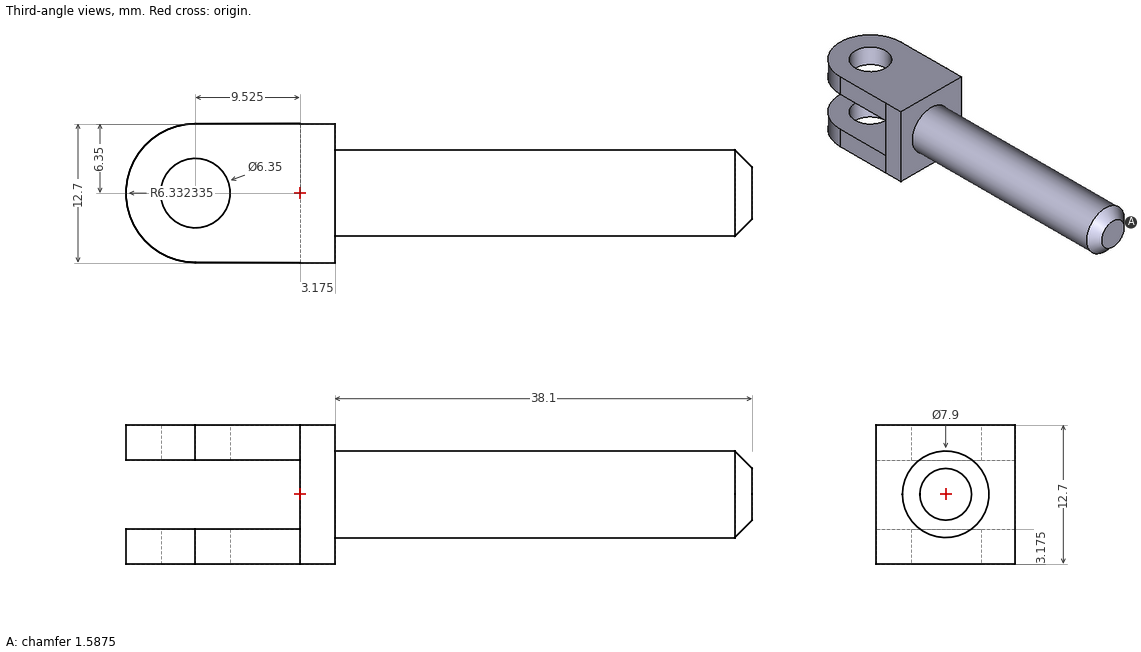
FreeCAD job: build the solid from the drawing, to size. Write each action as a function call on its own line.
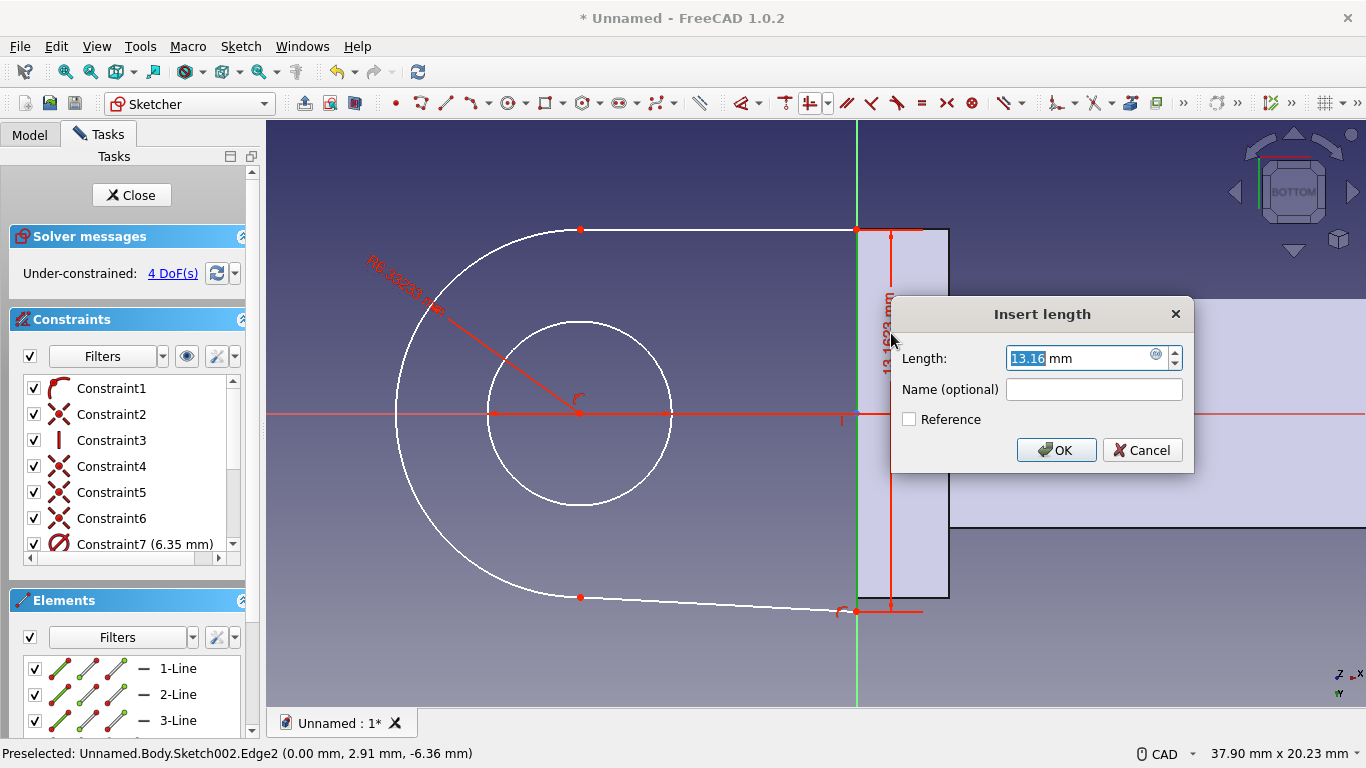
text(12.7)
key(Return)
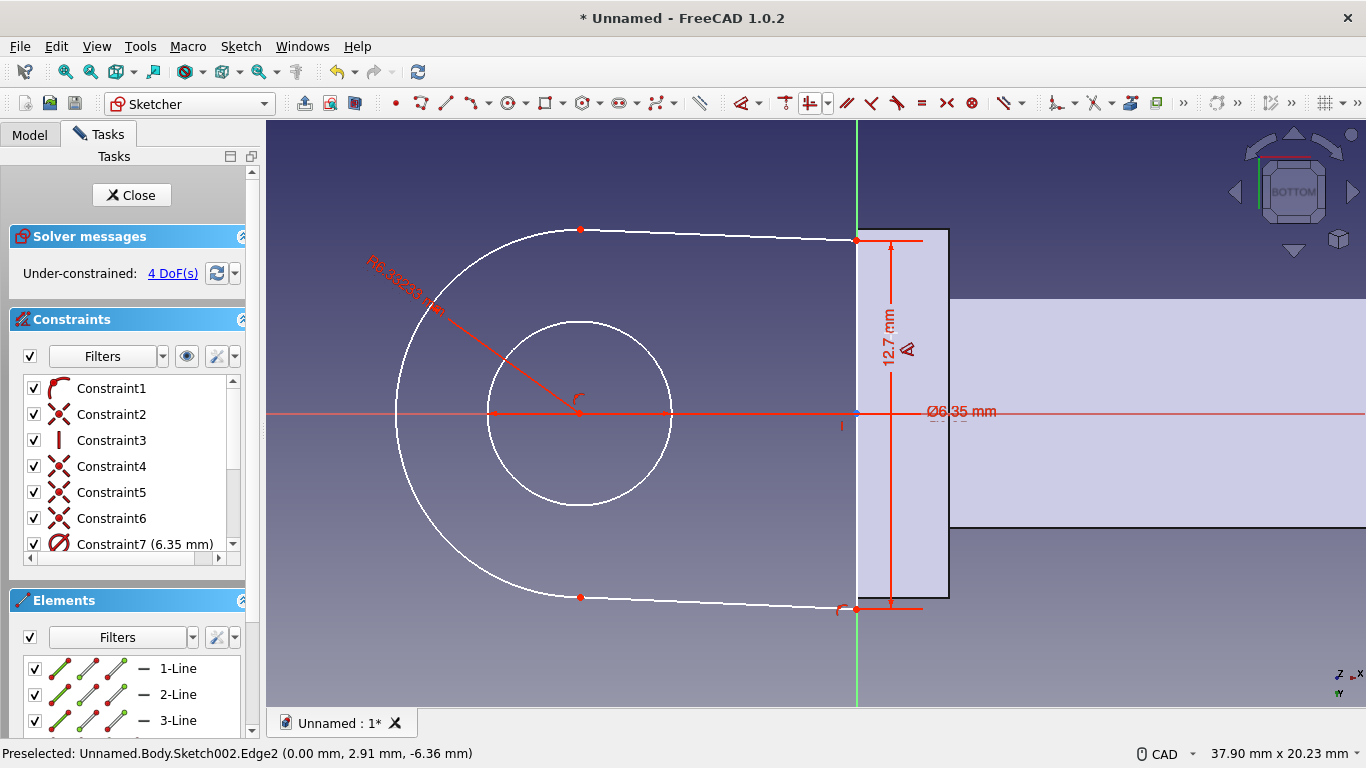
click(857, 609)
click(891, 511)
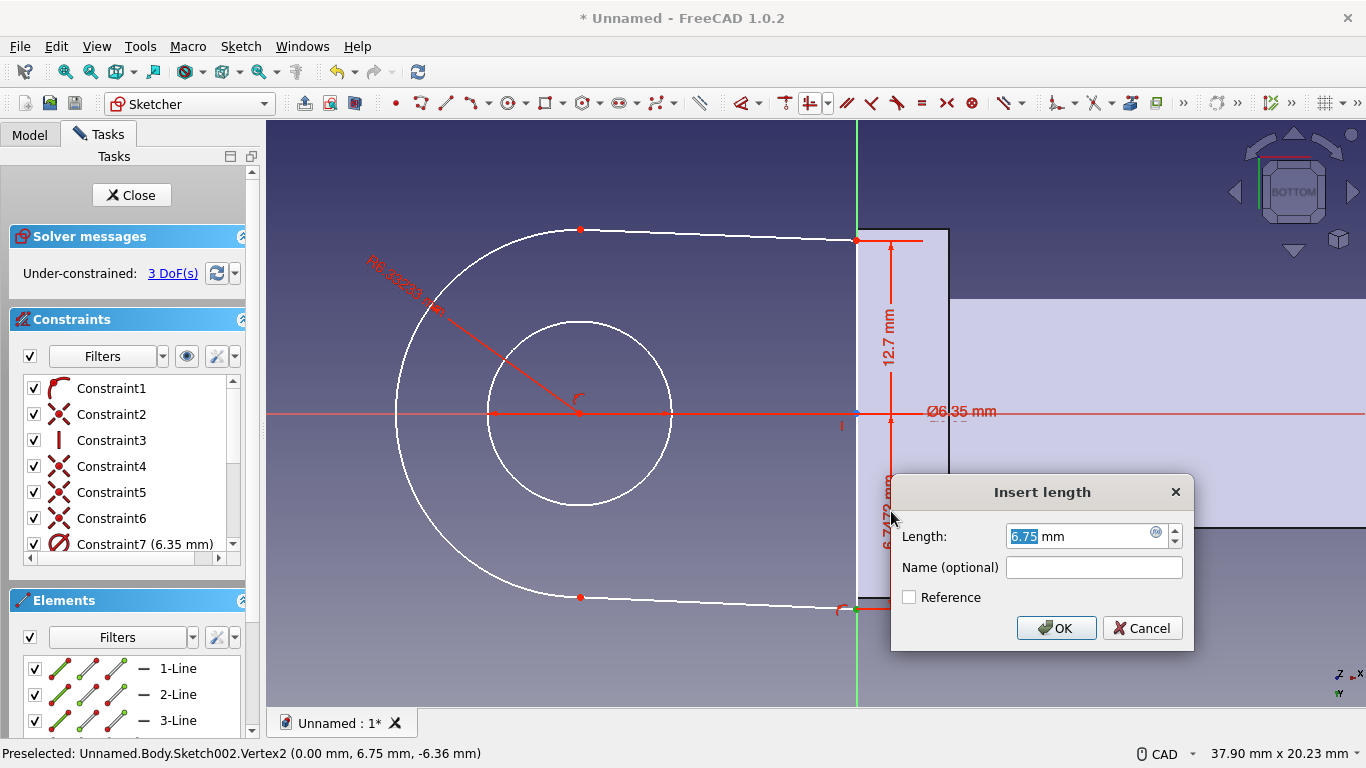
text(6.35)
key(Return)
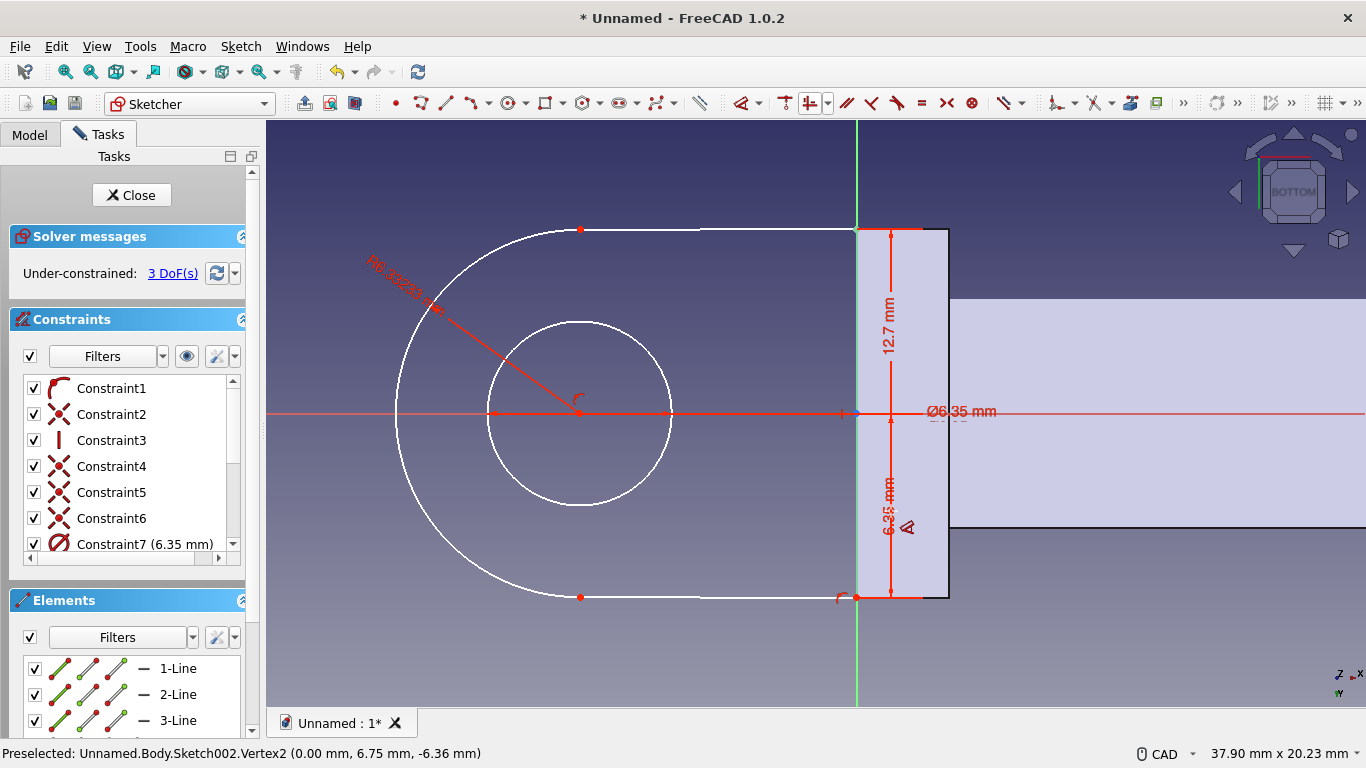
click(580, 414)
click(718, 448)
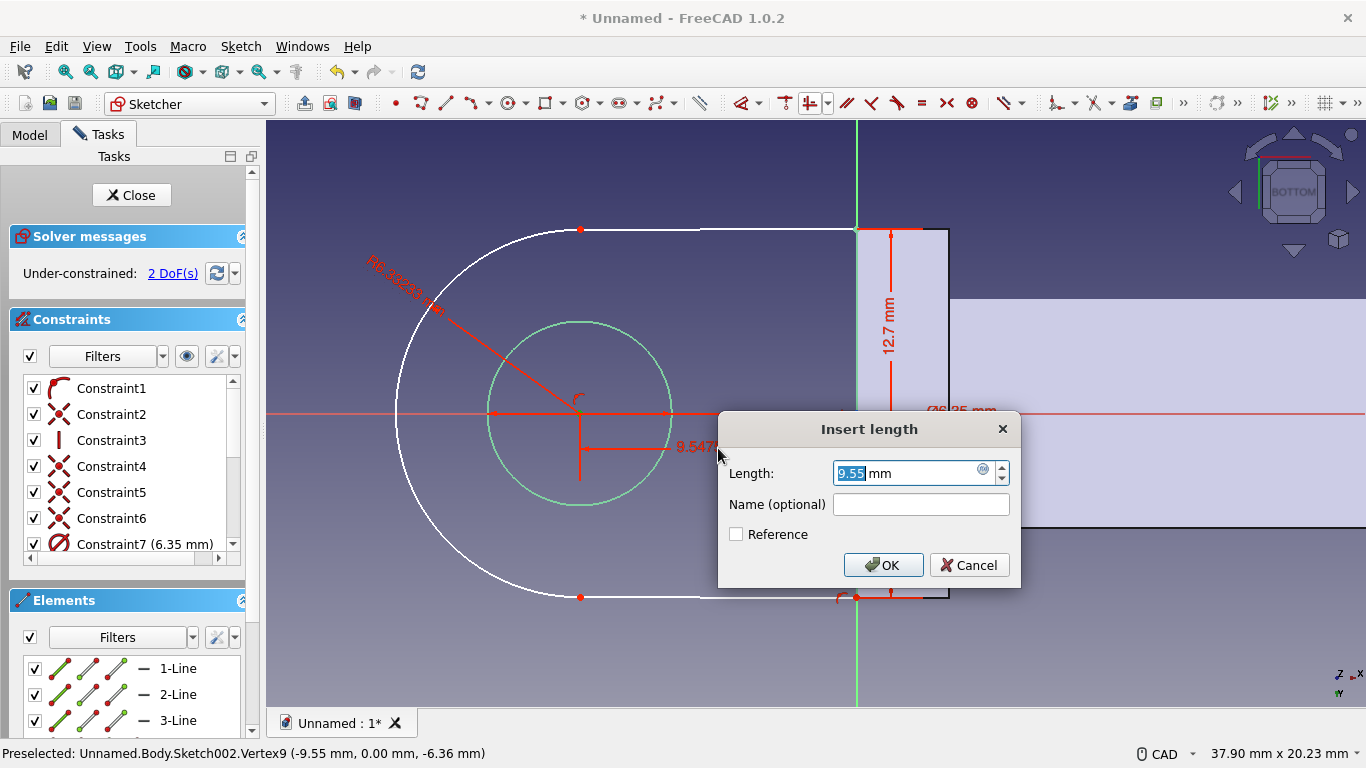
text(9.525)
key(Return)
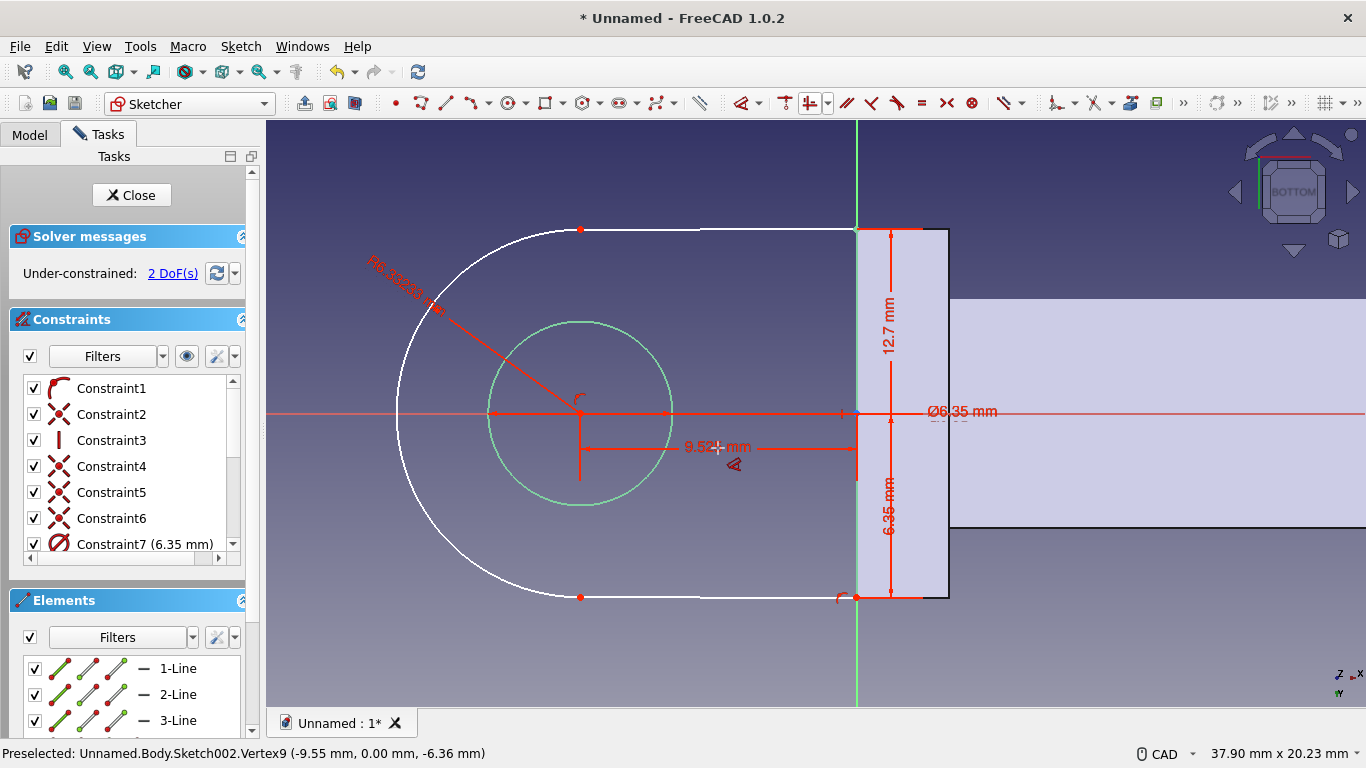
click(580, 597)
click(718, 631)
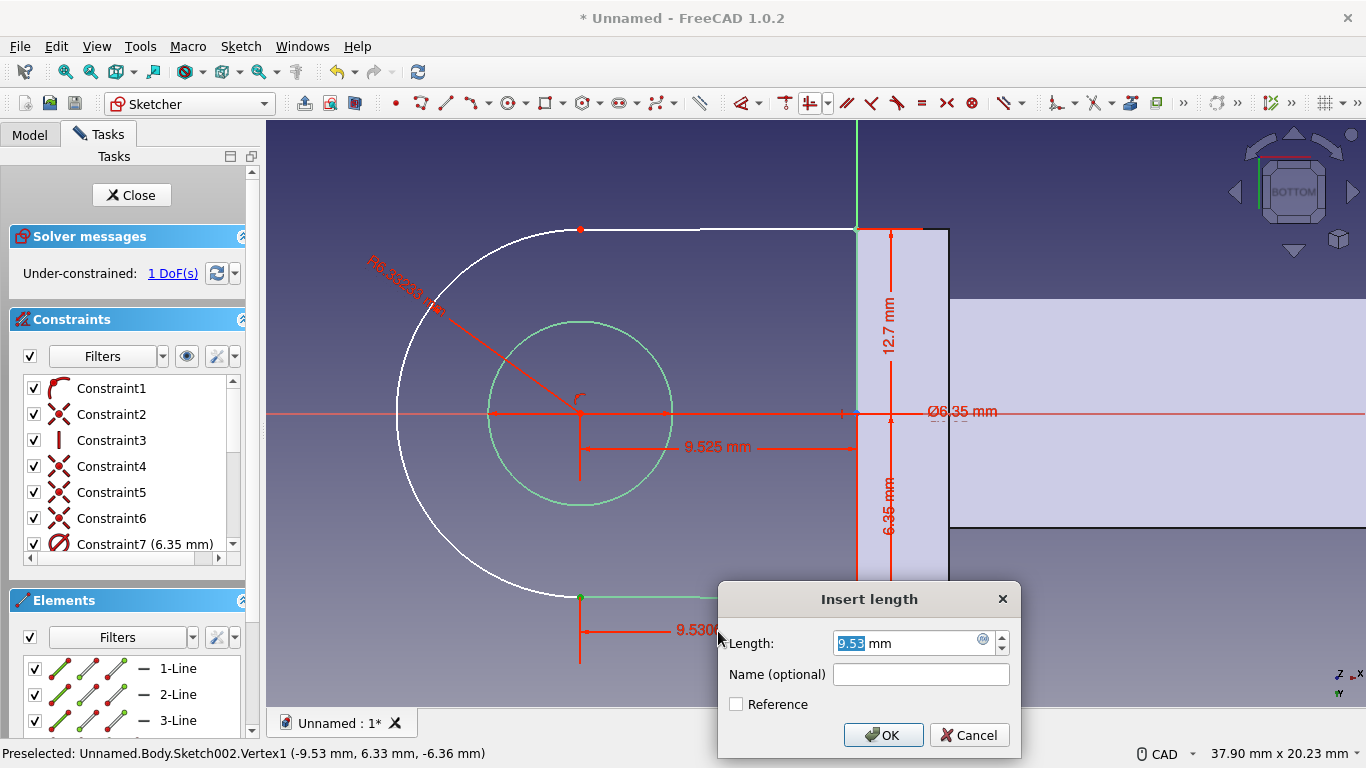
text(9.525)
key(Return)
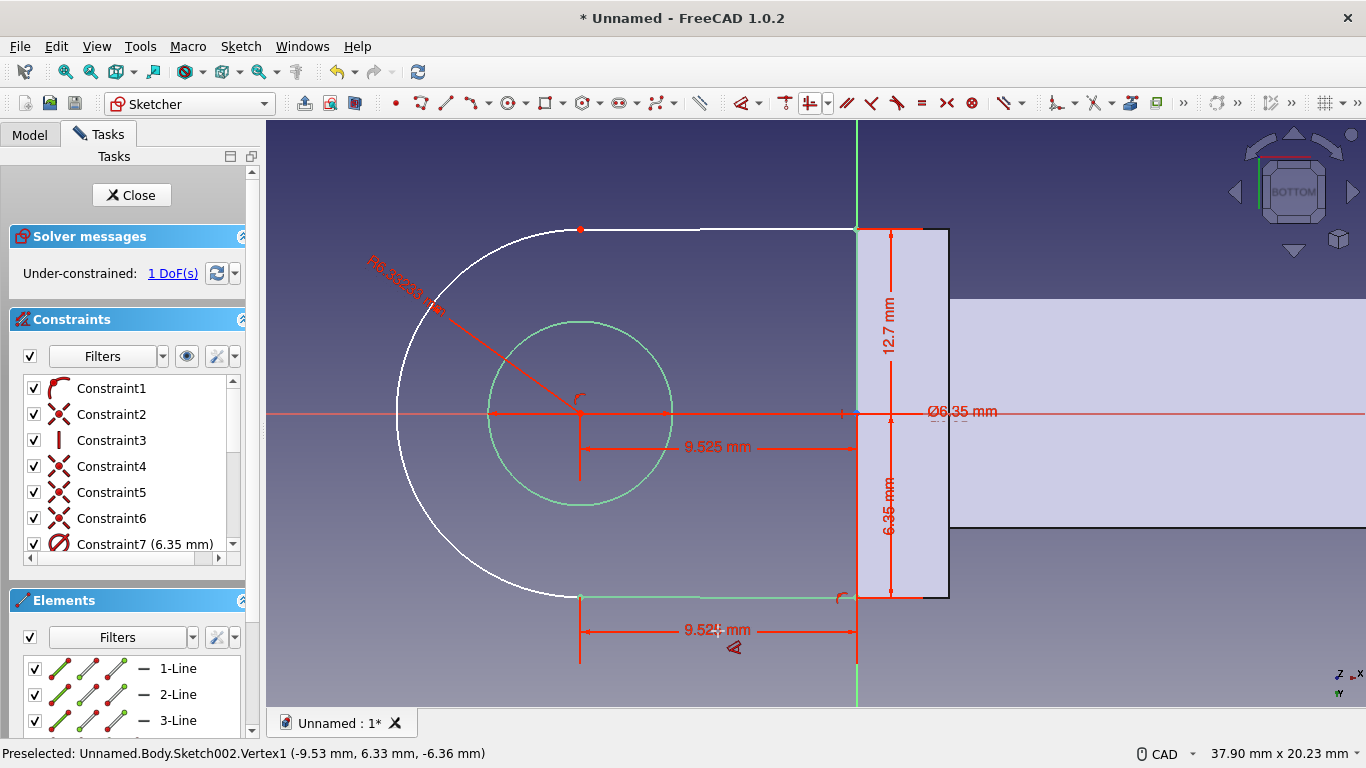
click(580, 230)
click(718, 196)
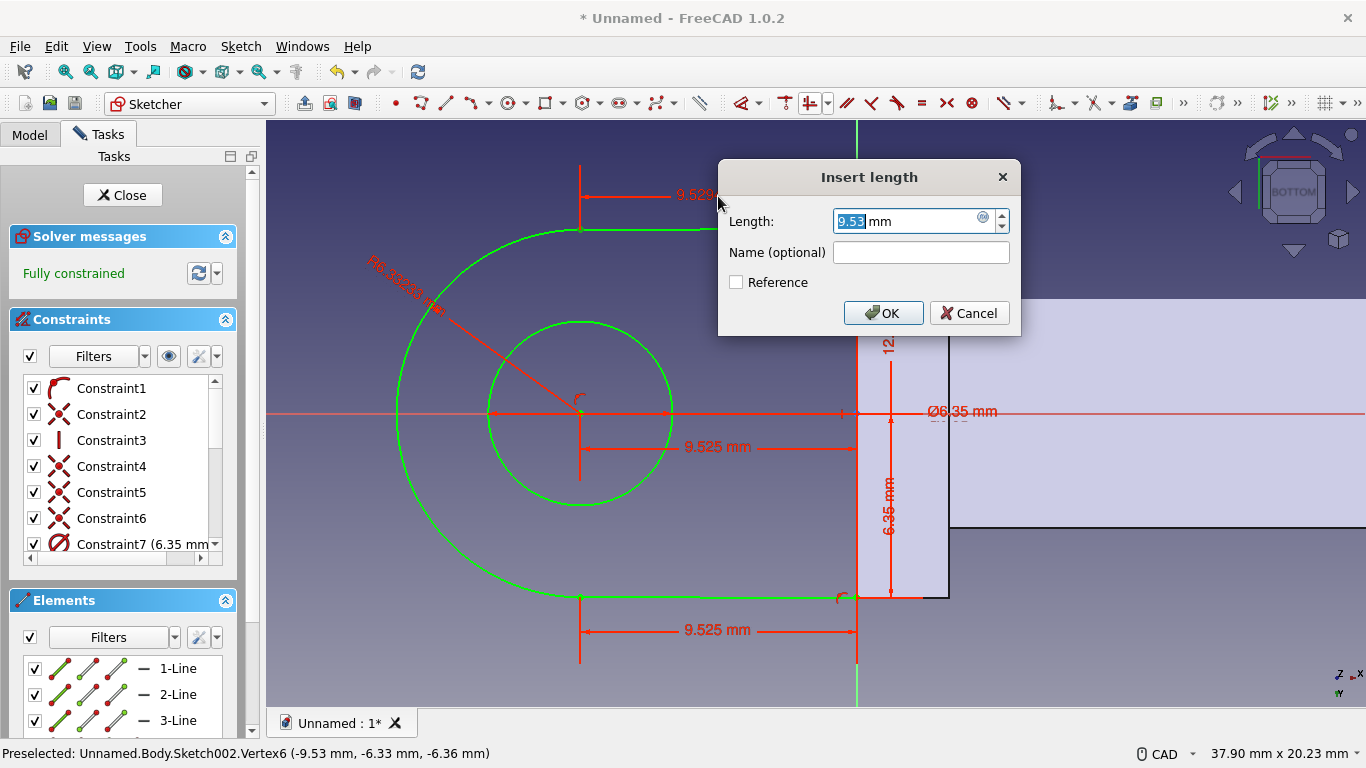
text(9.525)
key(Return)
key(Escape)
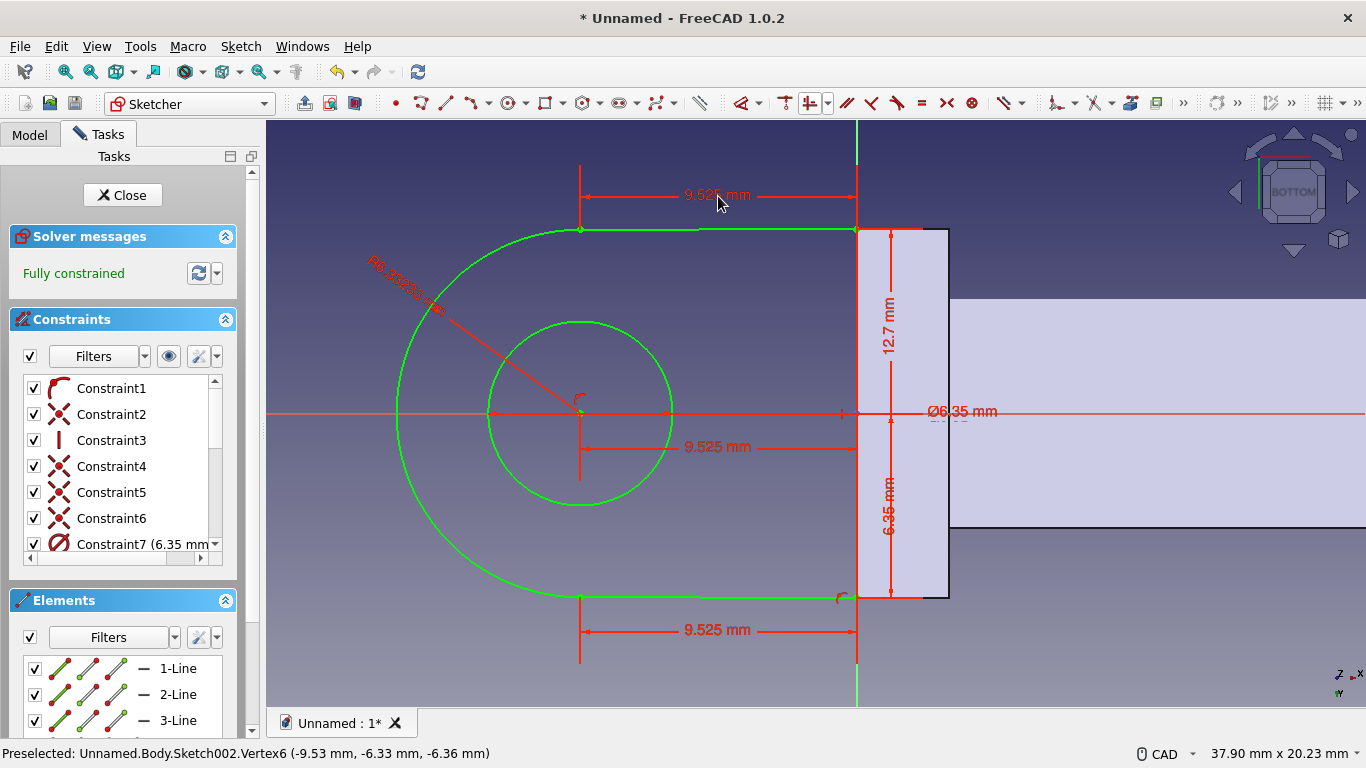
click(123, 195)